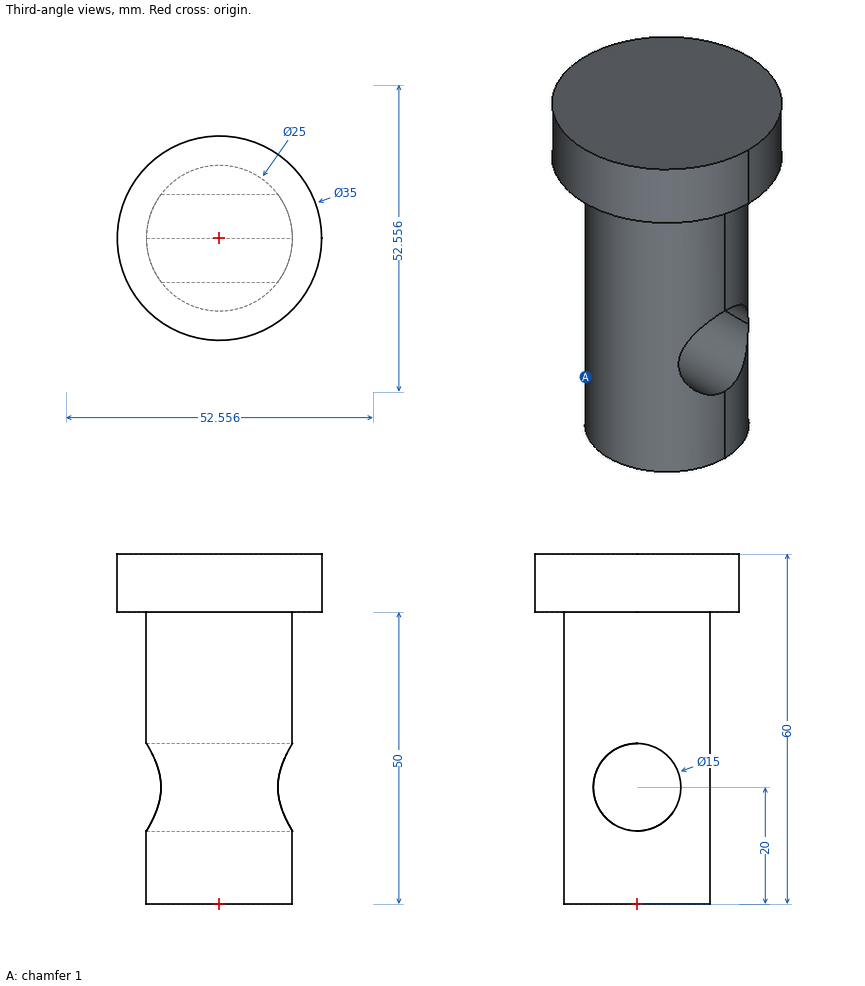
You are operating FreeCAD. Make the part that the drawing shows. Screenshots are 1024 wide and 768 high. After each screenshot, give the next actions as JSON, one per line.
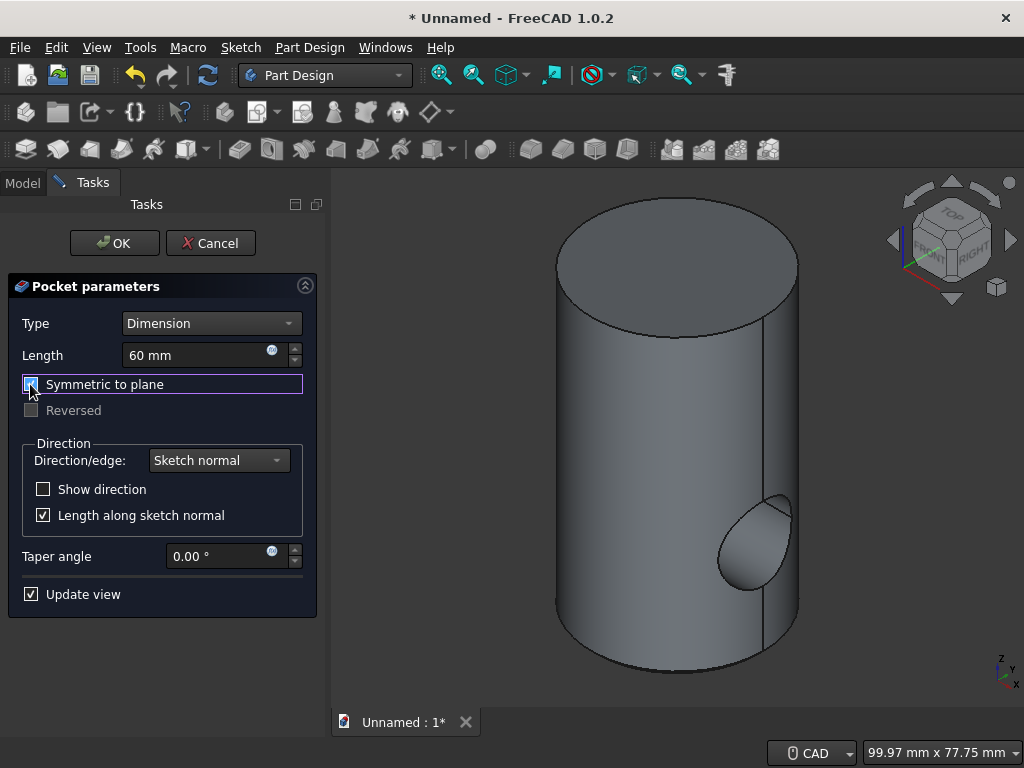
{"action": "left_click", "coordinate": [115, 243]}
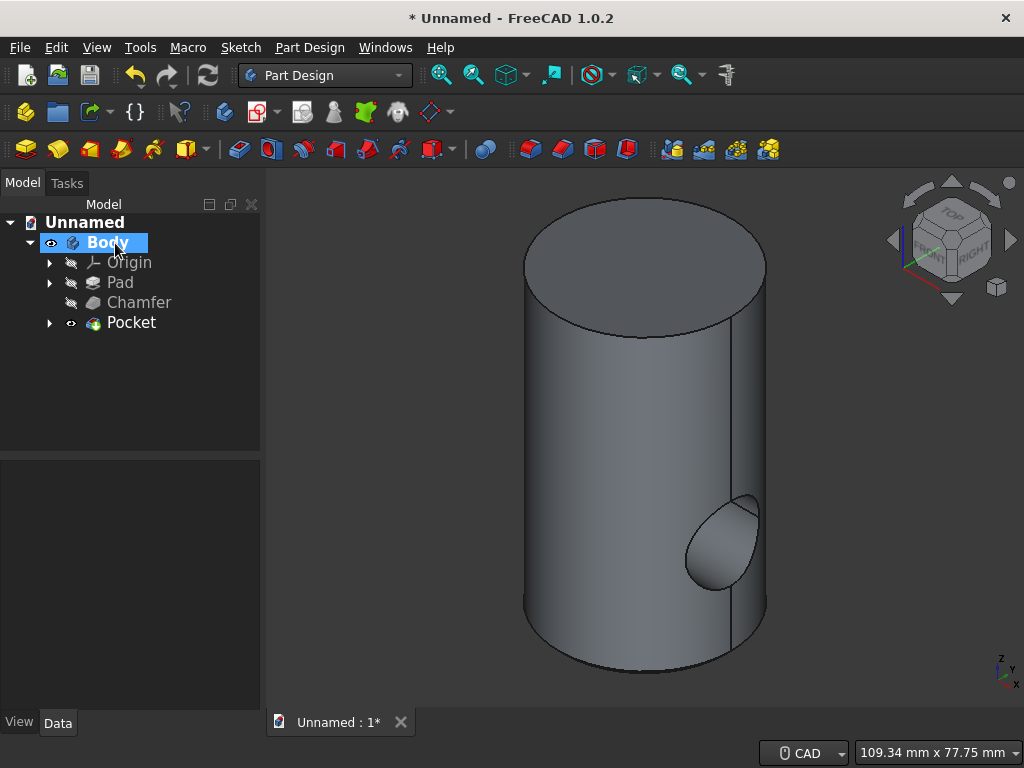
{"action": "left_click", "coordinate": [258, 112]}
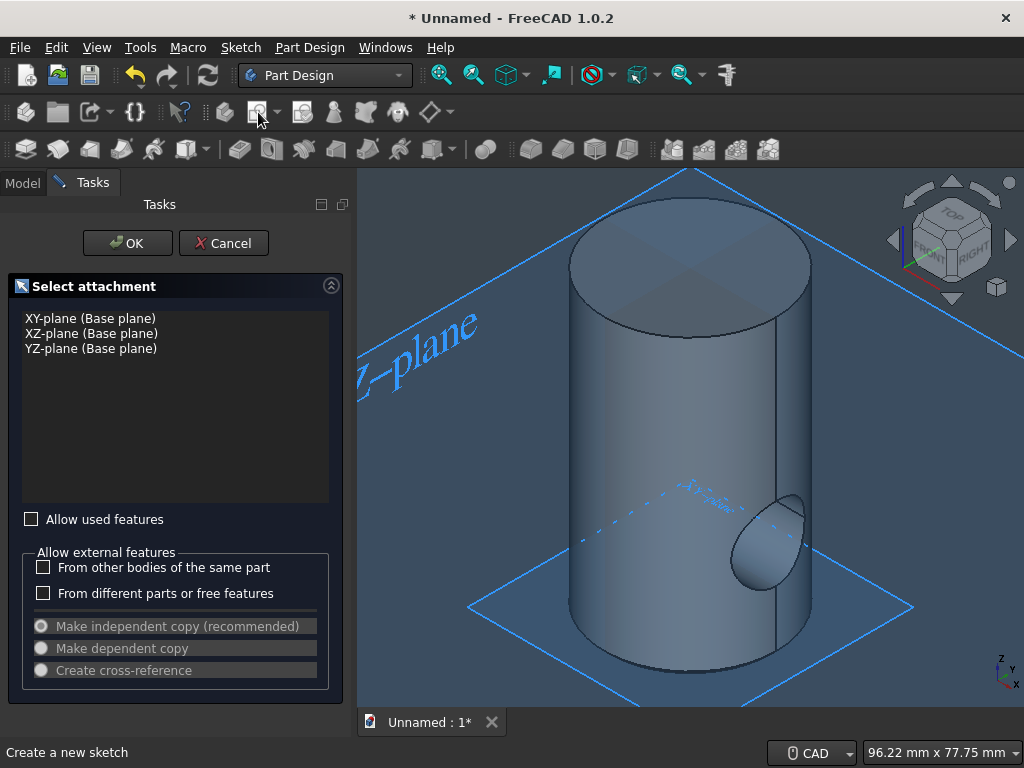
{"action": "left_click", "coordinate": [82, 318]}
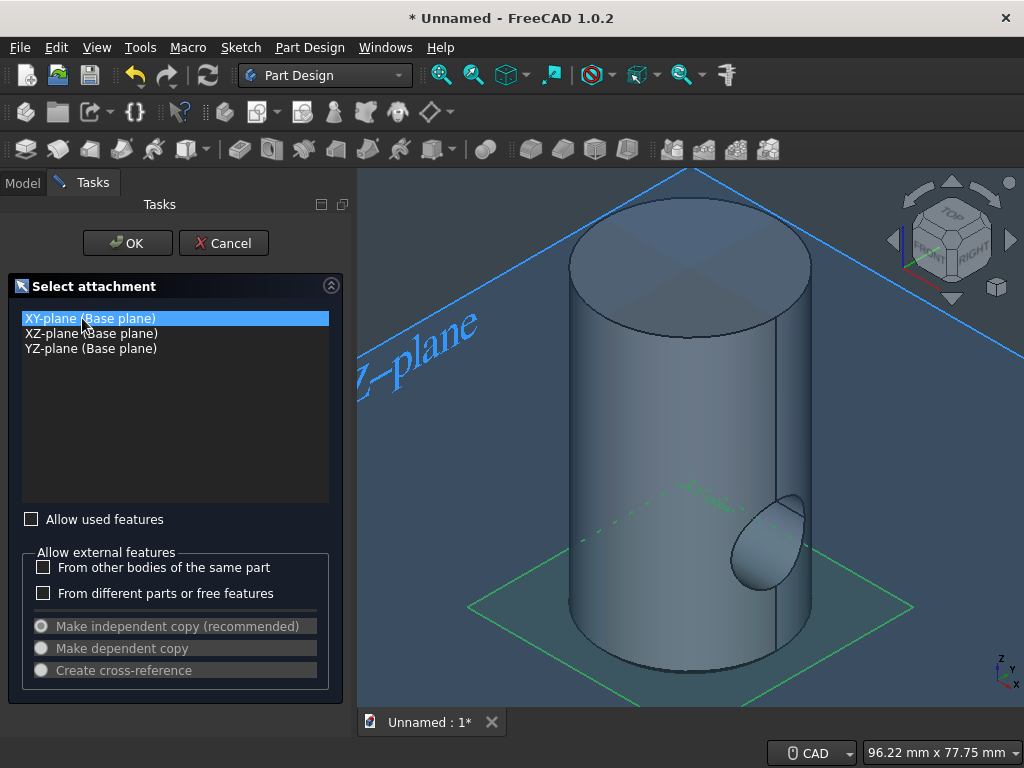
{"action": "left_click", "coordinate": [128, 243]}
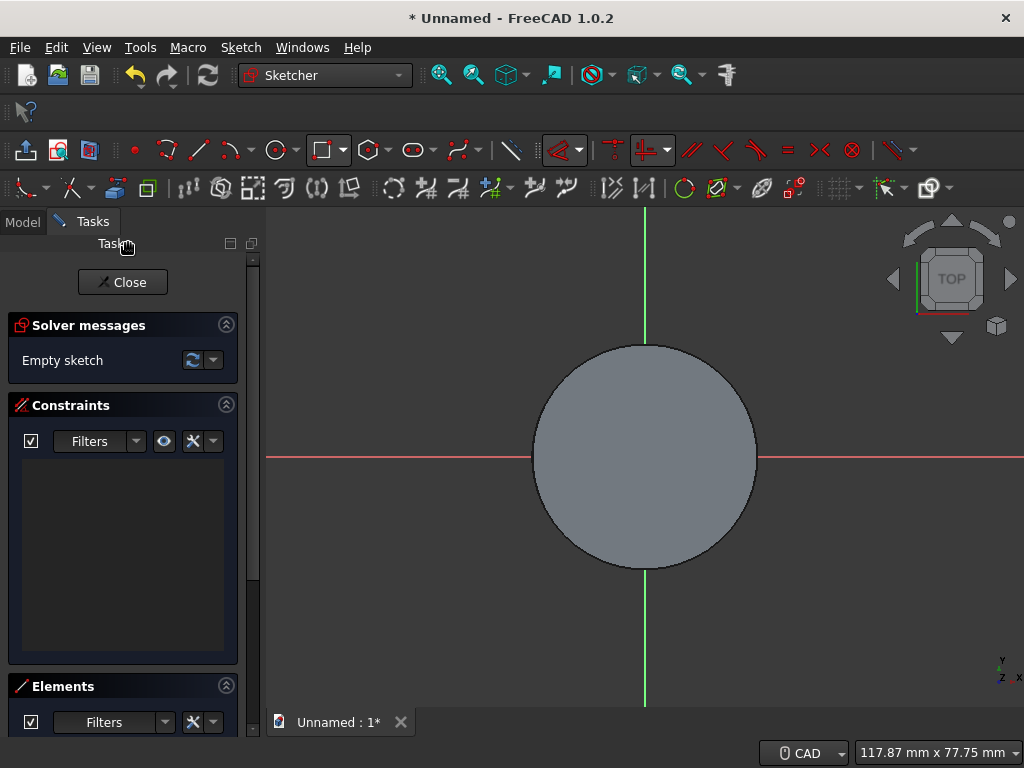
{"action": "left_click", "coordinate": [90, 150]}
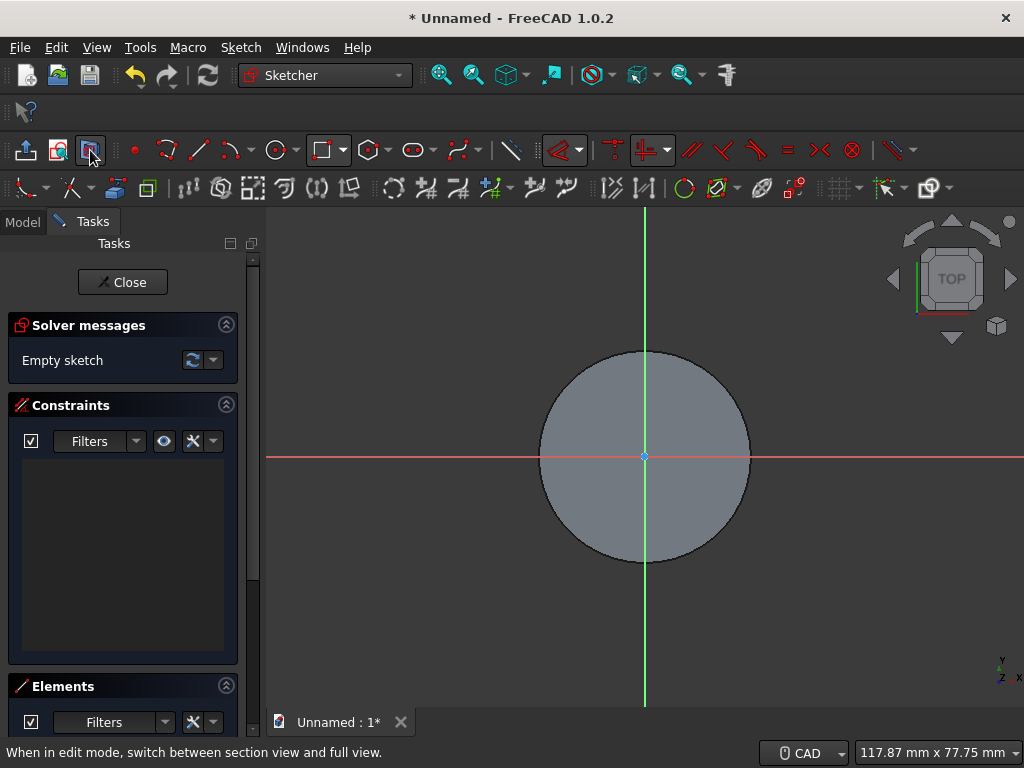
{"action": "key", "text": "g v"}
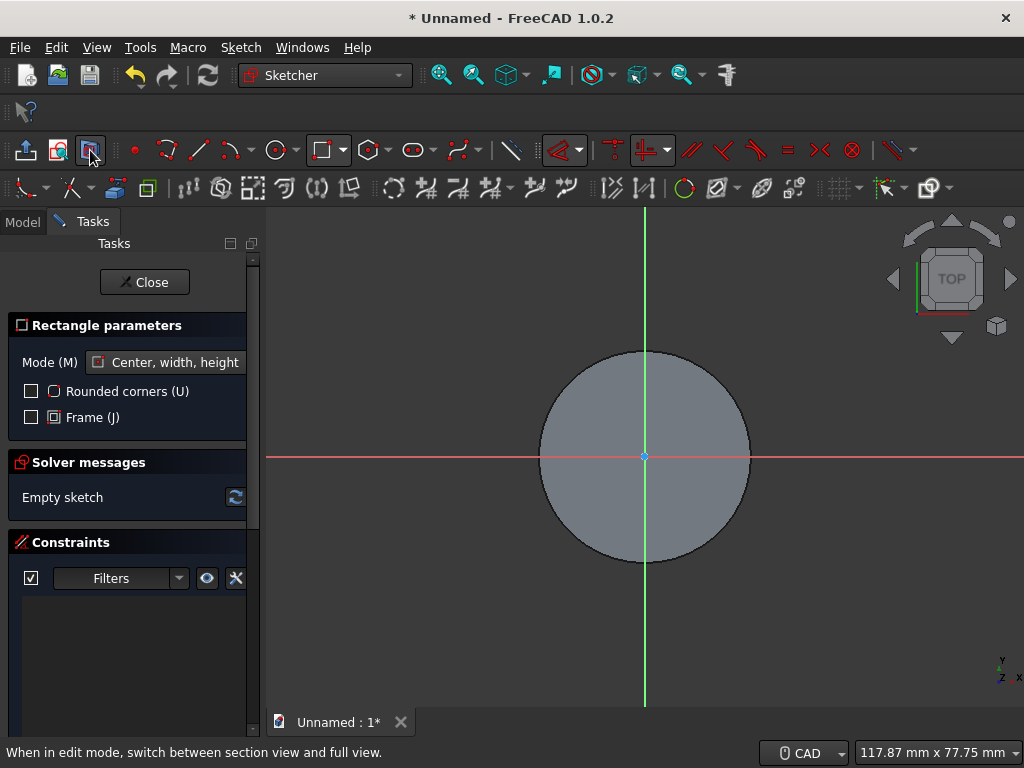
{"action": "left_click", "coordinate": [645, 457]}
{"action": "left_click", "coordinate": [814, 288]}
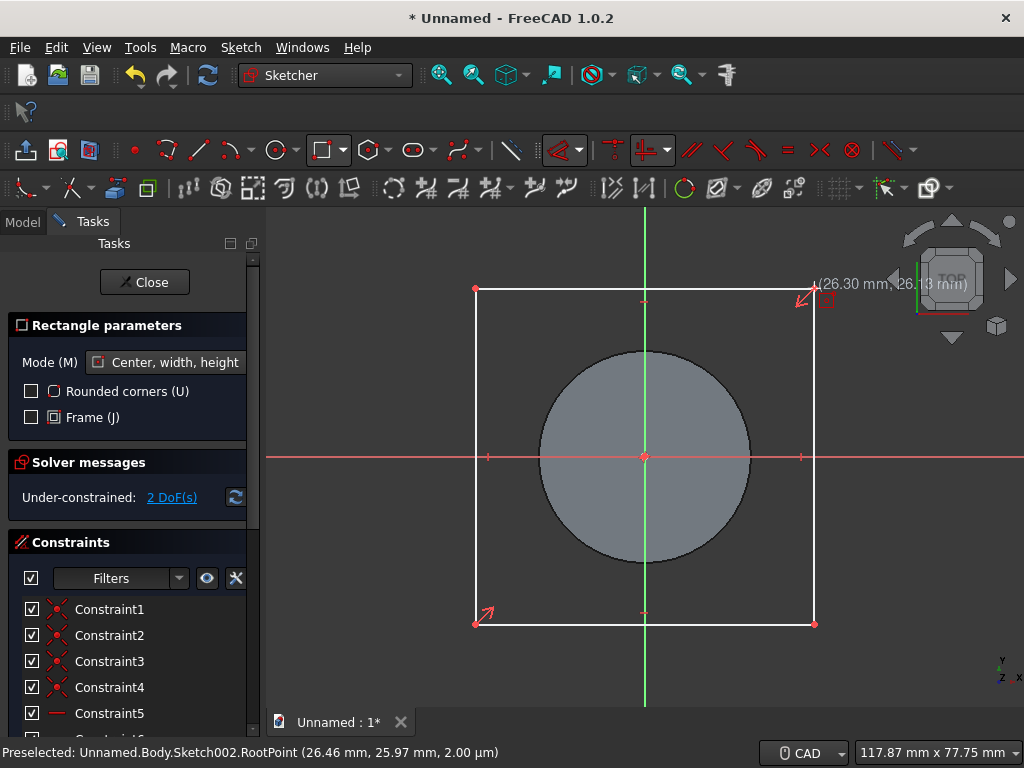
{"action": "left_click", "coordinate": [276, 150]}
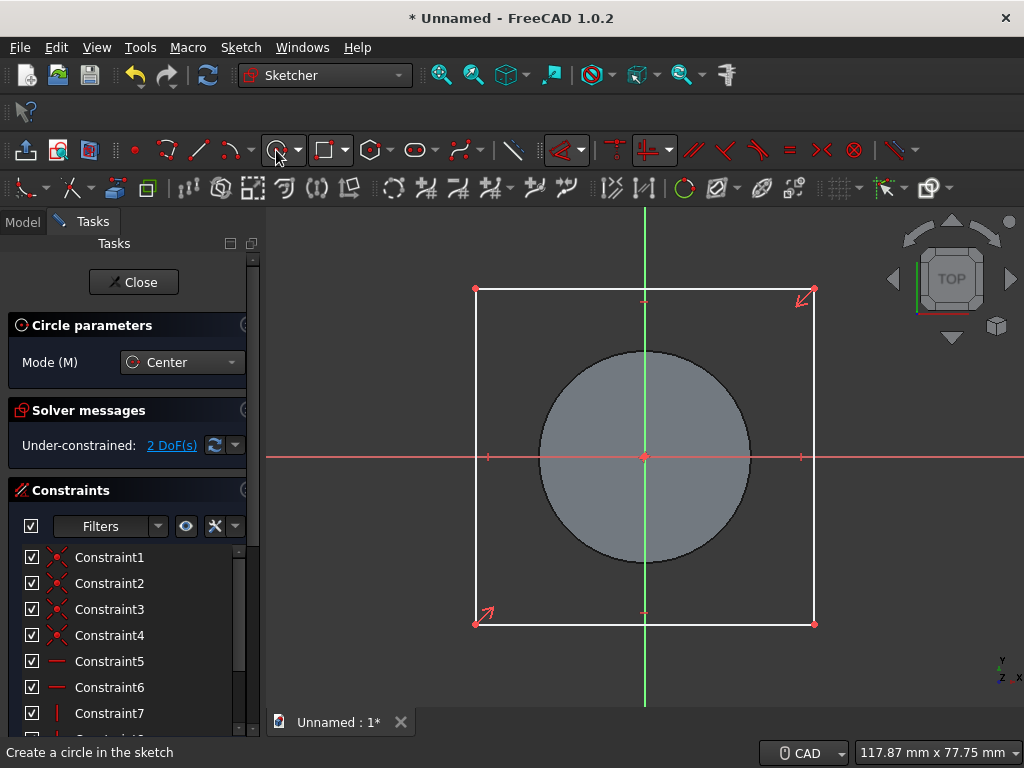
{"action": "left_click", "coordinate": [645, 457]}
{"action": "left_click", "coordinate": [702, 400]}
{"action": "key", "text": "Escape"}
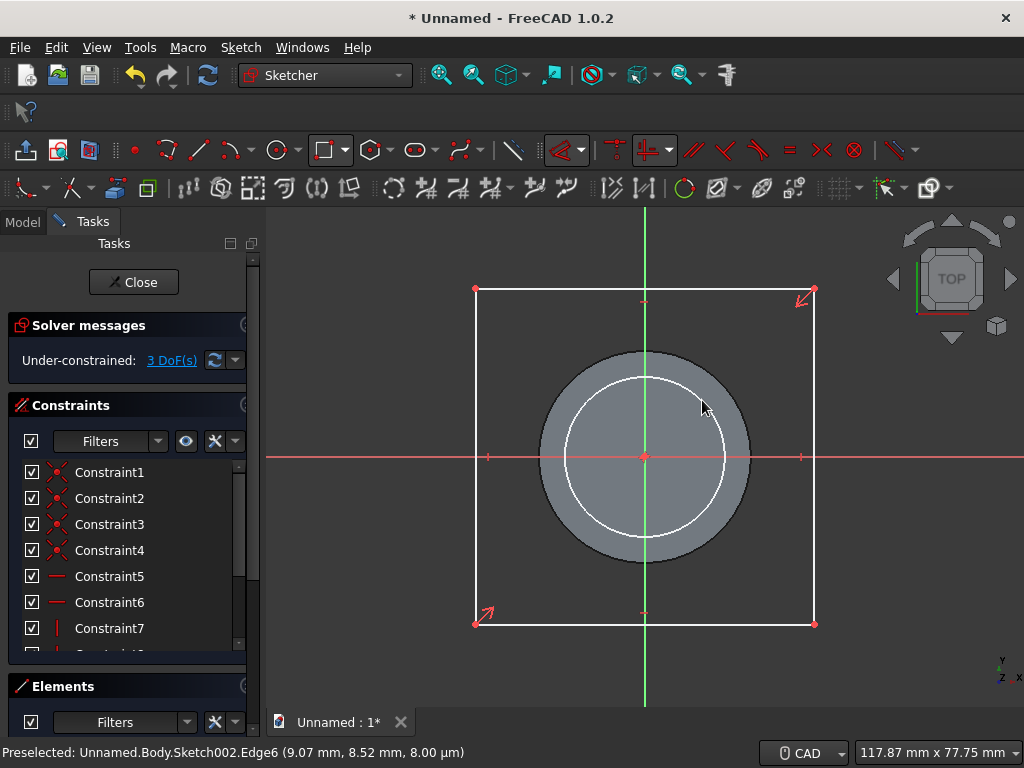
{"action": "left_click", "coordinate": [701, 400]}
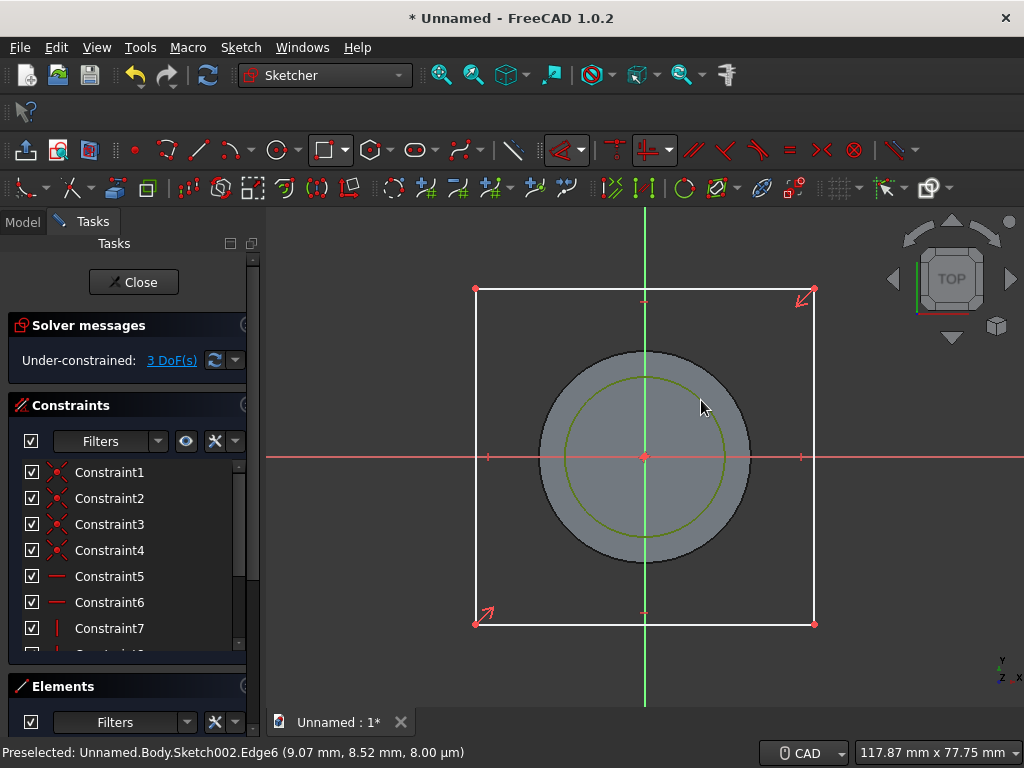
{"action": "left_click", "coordinate": [584, 150]}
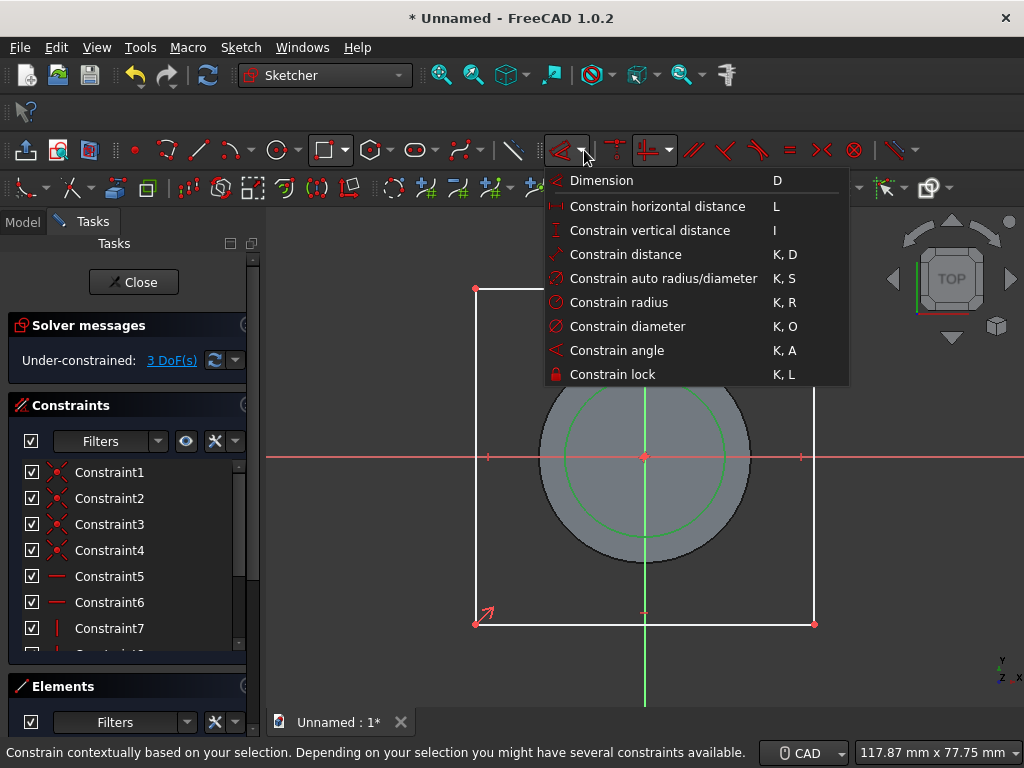
{"action": "left_click", "coordinate": [697, 326]}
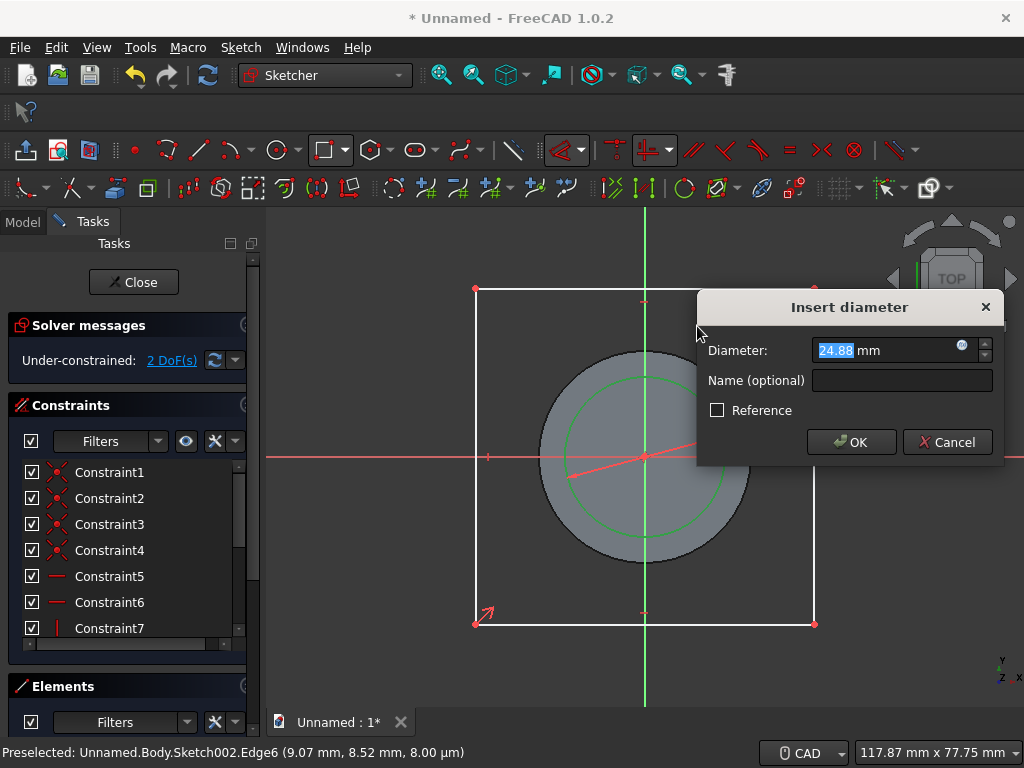
{"action": "type", "text": "25"}
{"action": "key", "text": "Return"}